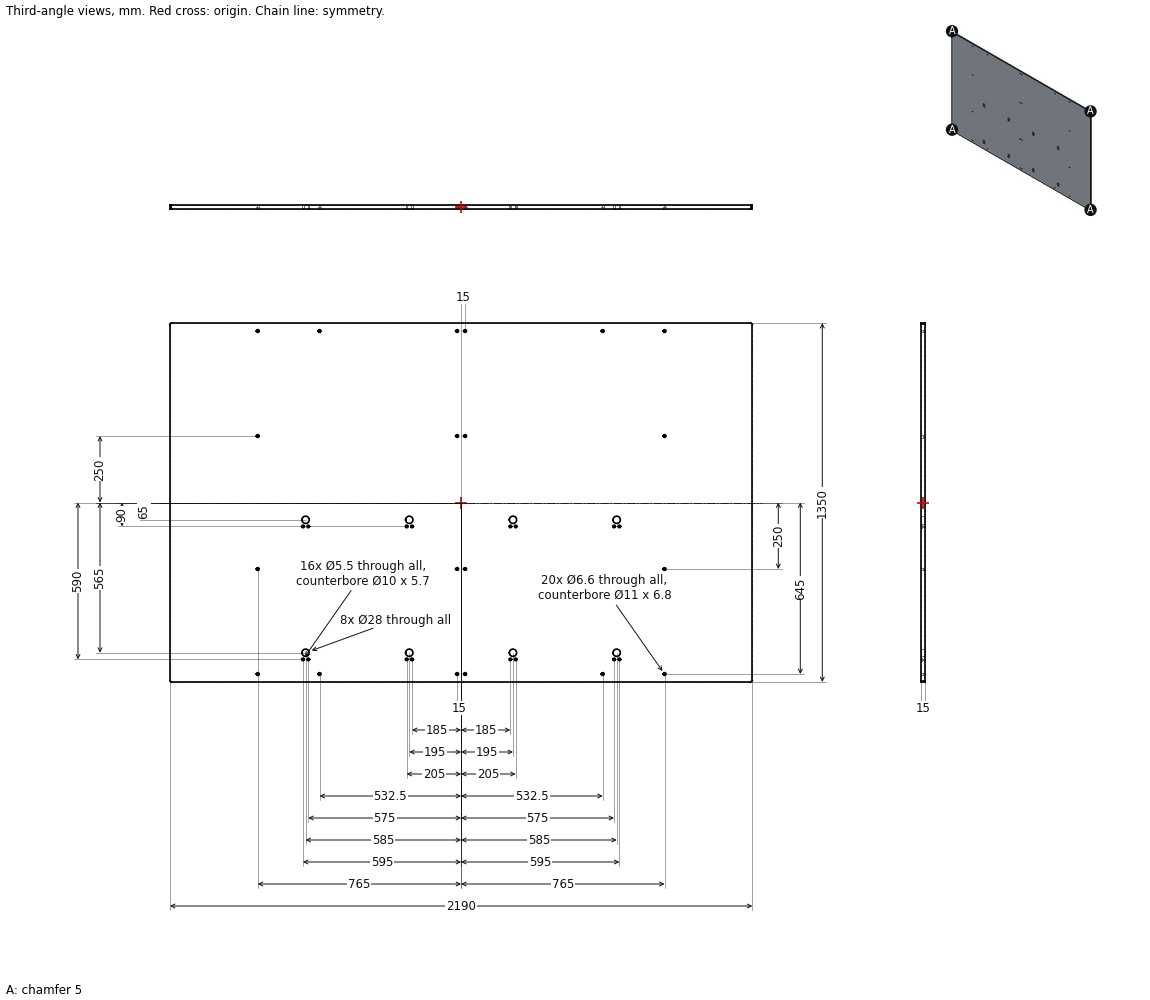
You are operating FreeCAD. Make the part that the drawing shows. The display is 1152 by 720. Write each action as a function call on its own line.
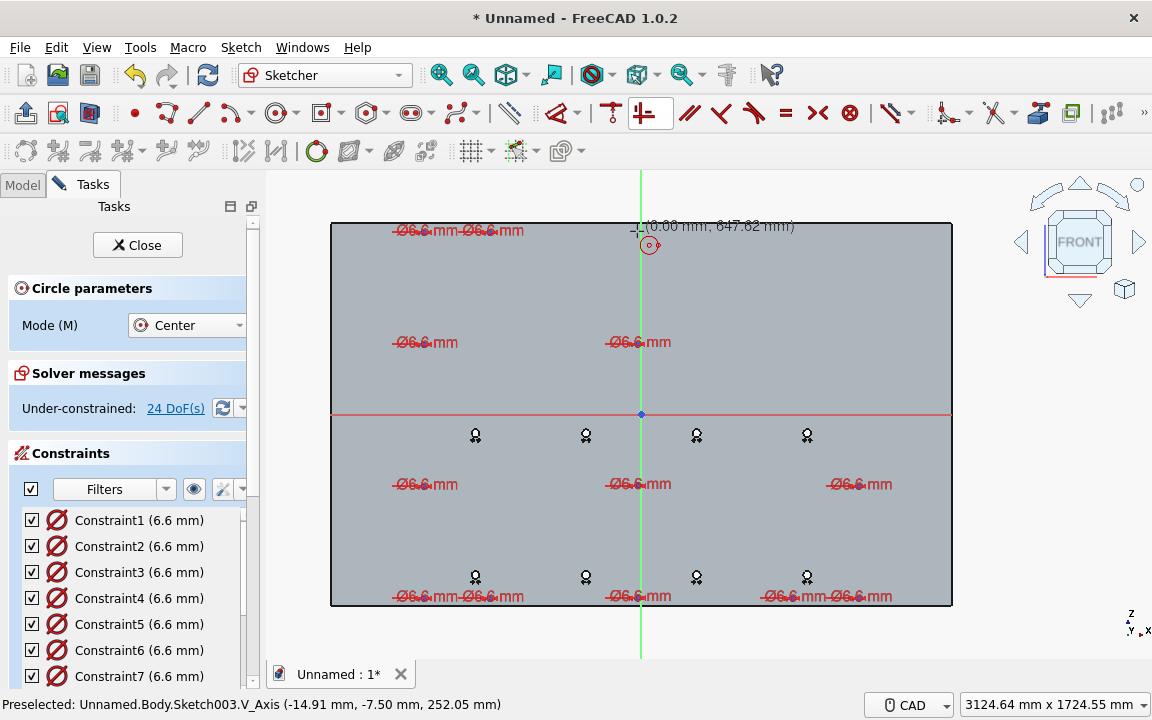
scroll(637, 232, up, 7)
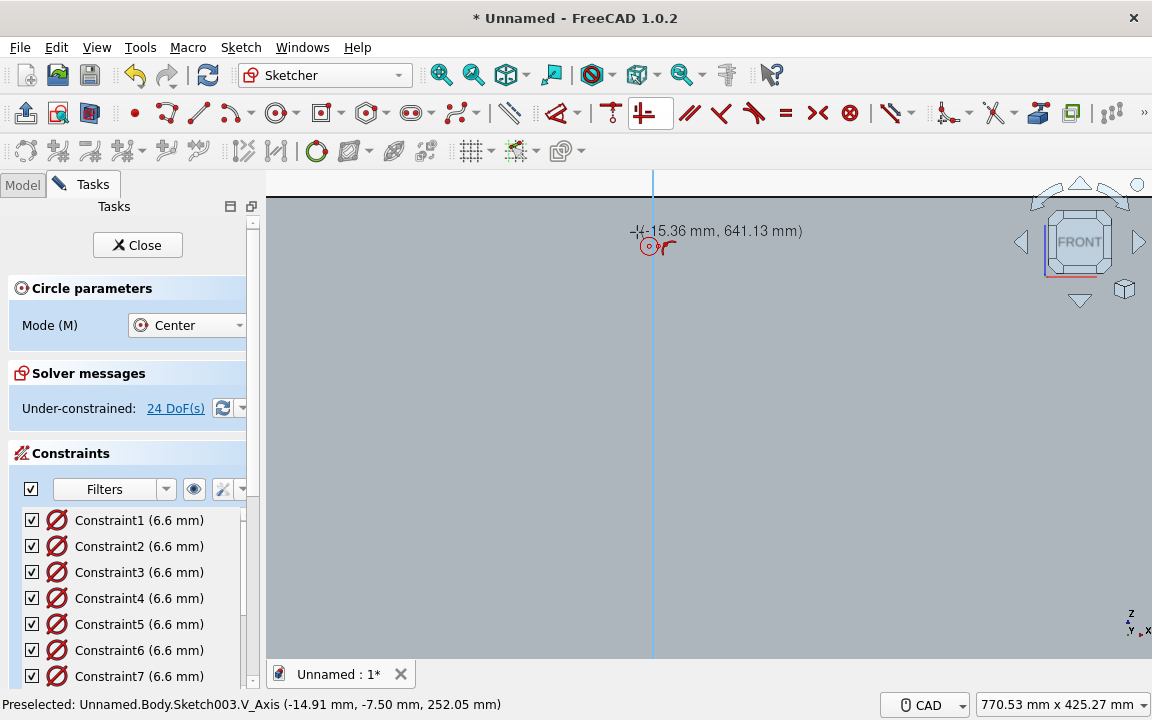
click(636, 231)
move(639, 229)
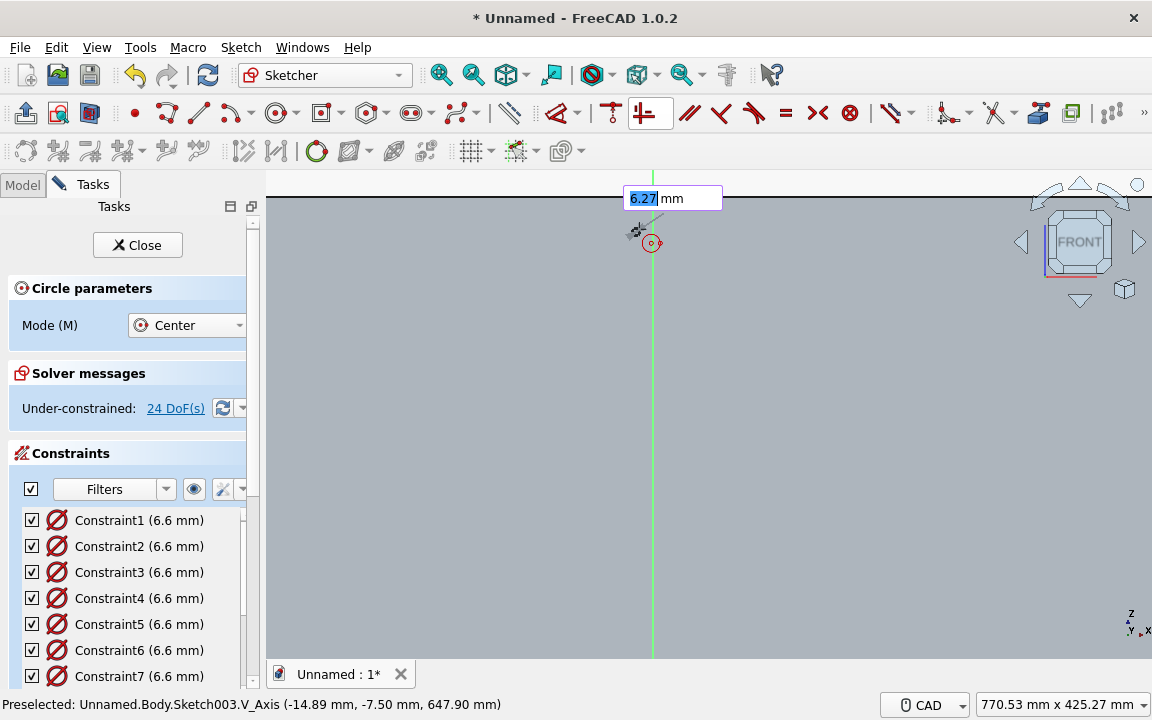
text(6.6)
key(Return)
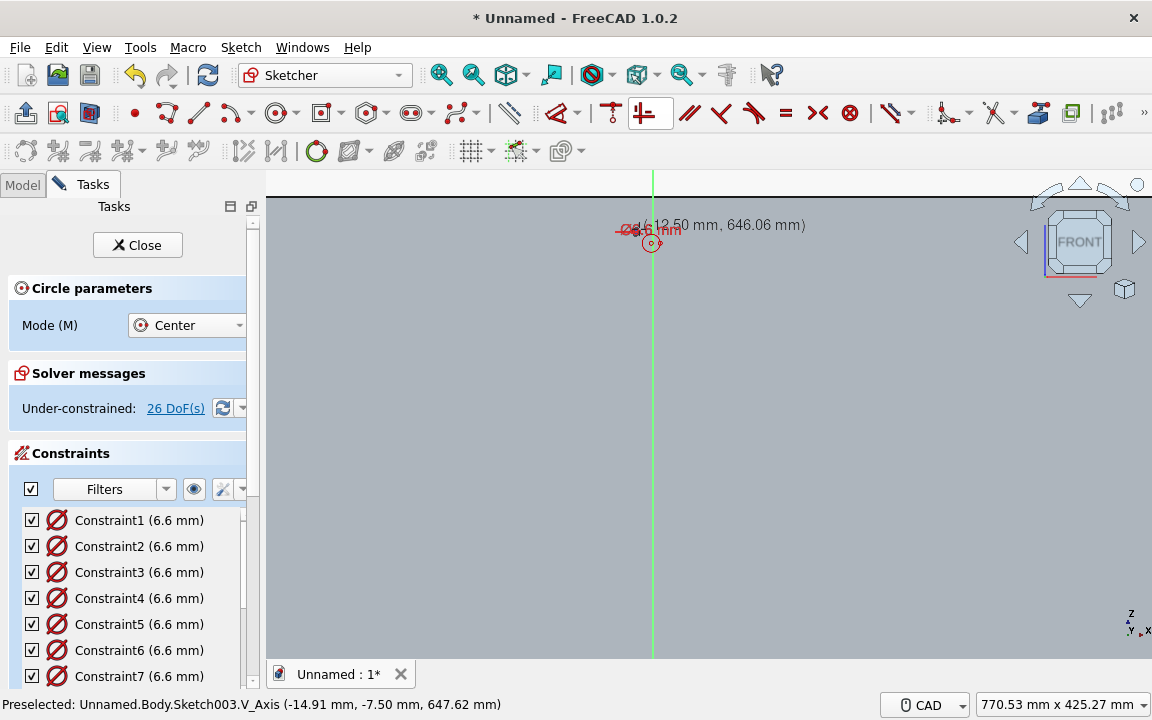
scroll(637, 273, down, 8)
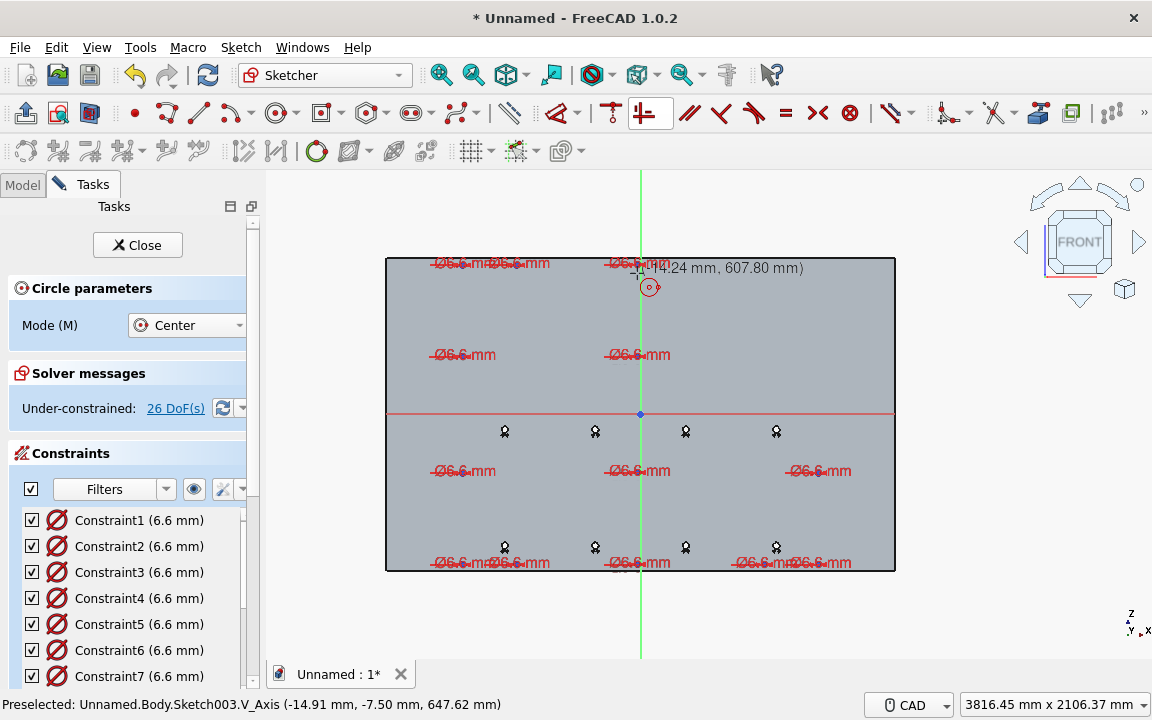
scroll(818, 356, up, 17)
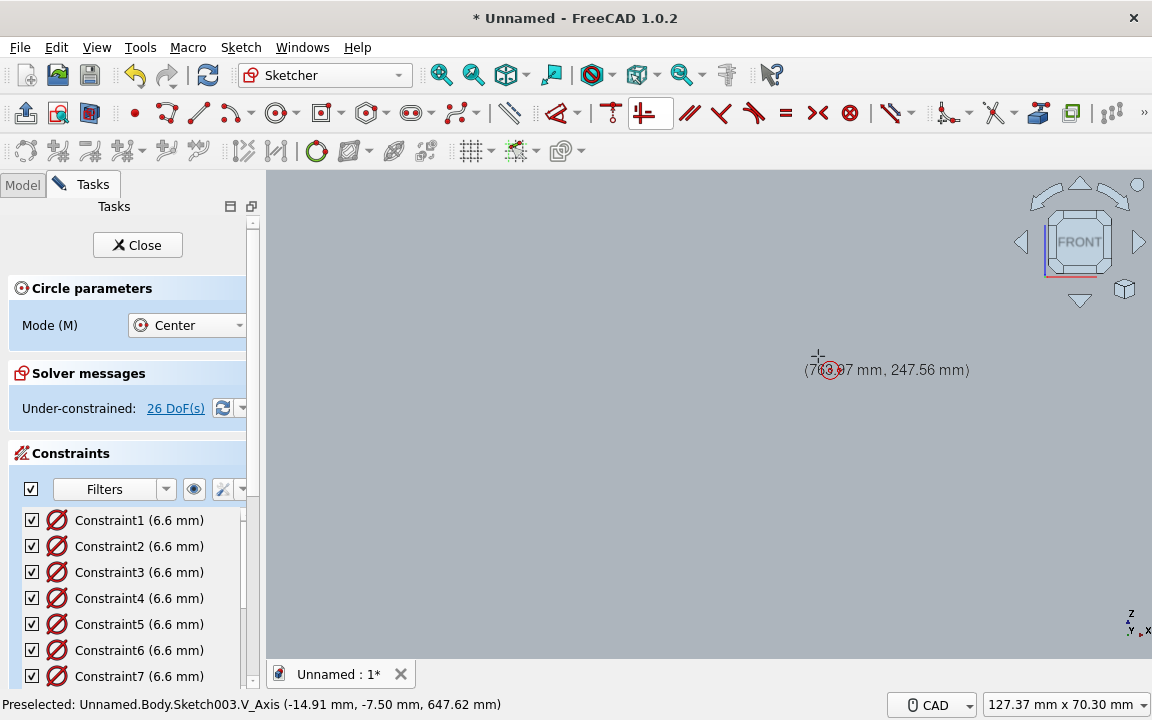
scroll(860, 343, down, 16)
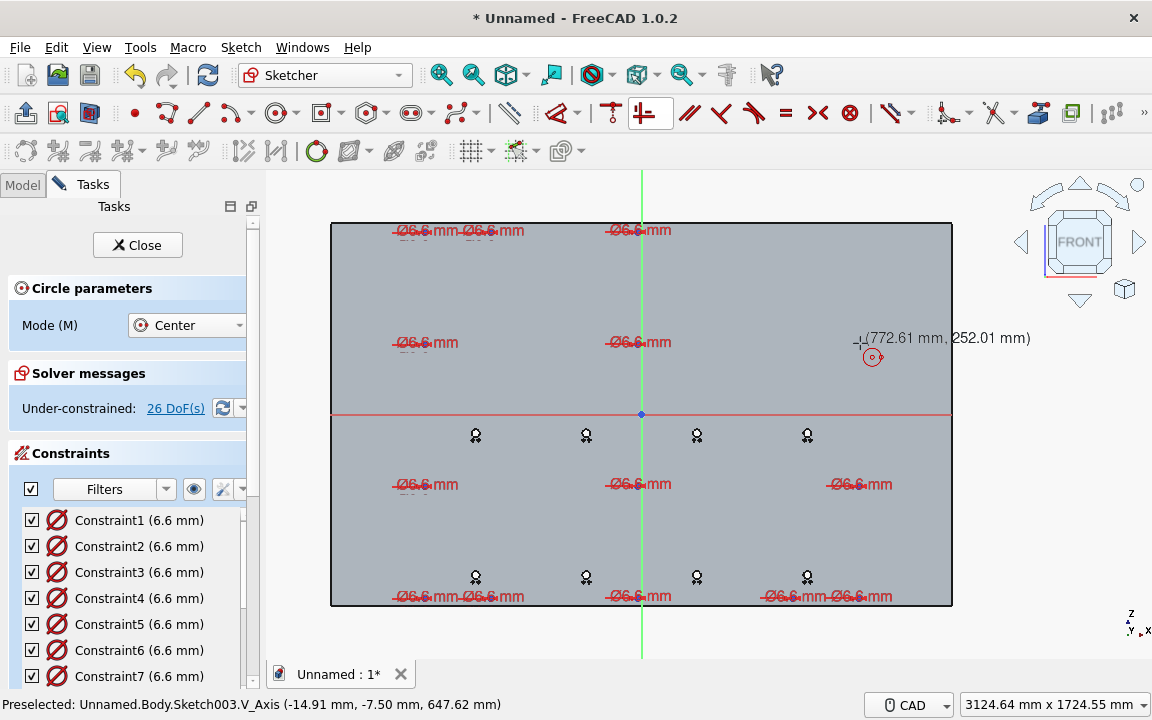
click(858, 344)
move(859, 343)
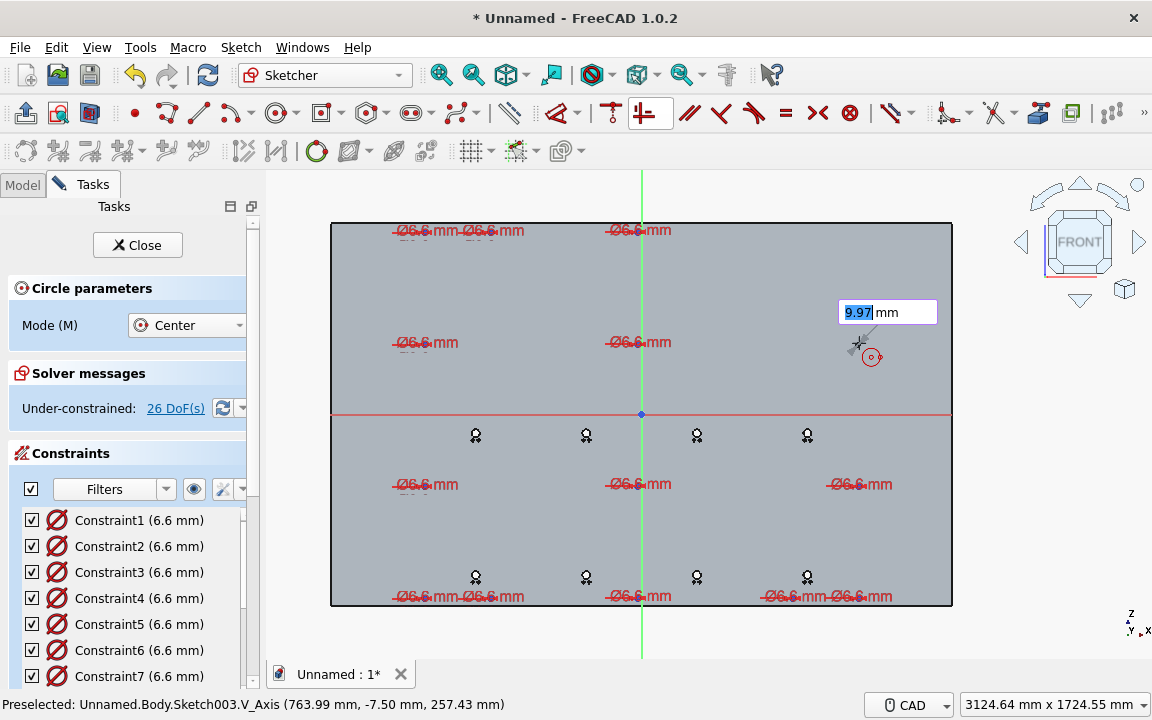
text(6.6)
key(Return)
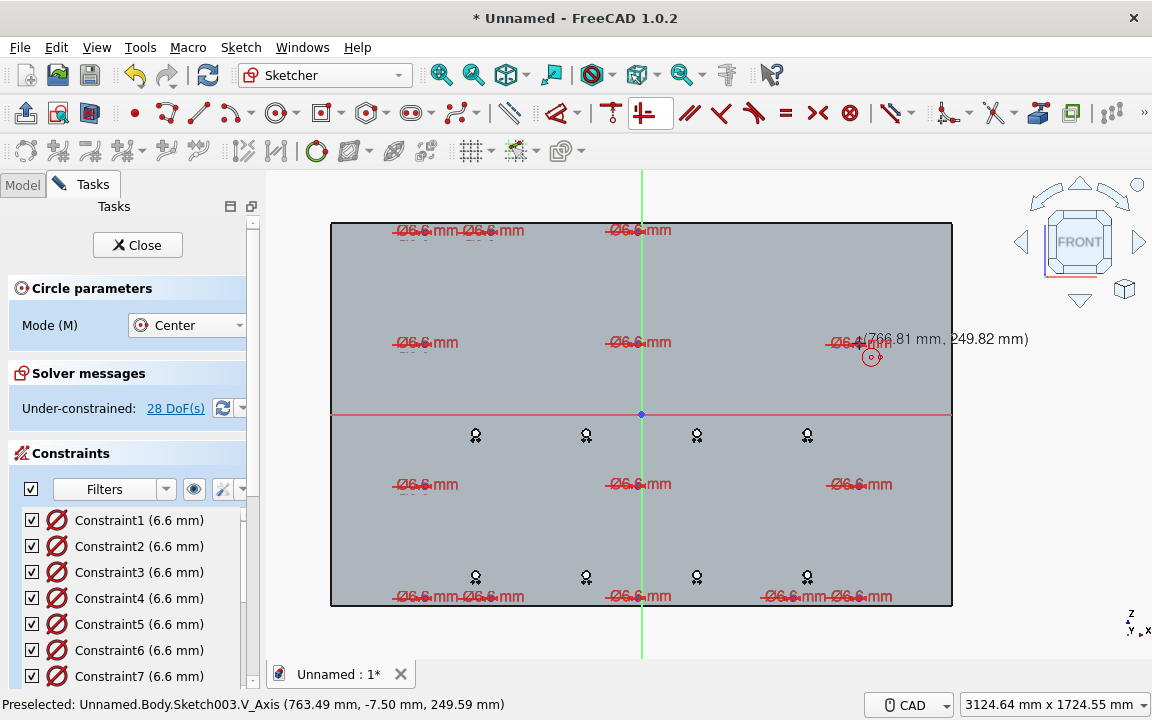
scroll(793, 232, up, 16)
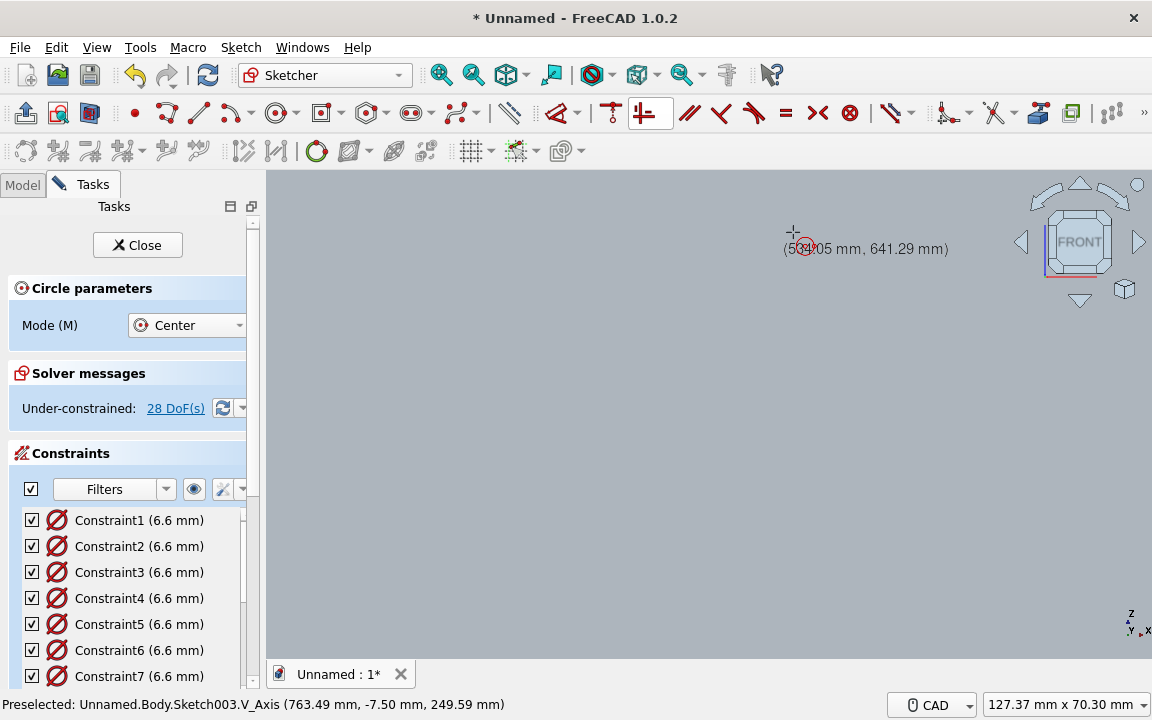
scroll(792, 232, down, 16)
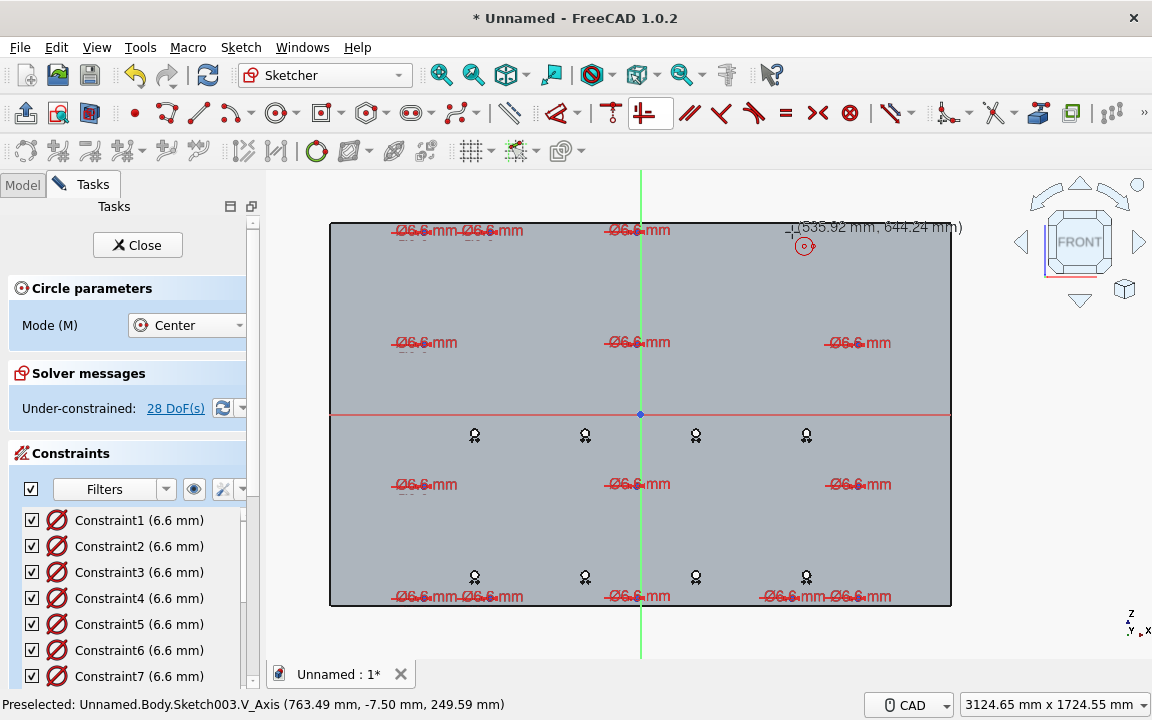
click(792, 232)
move(792, 231)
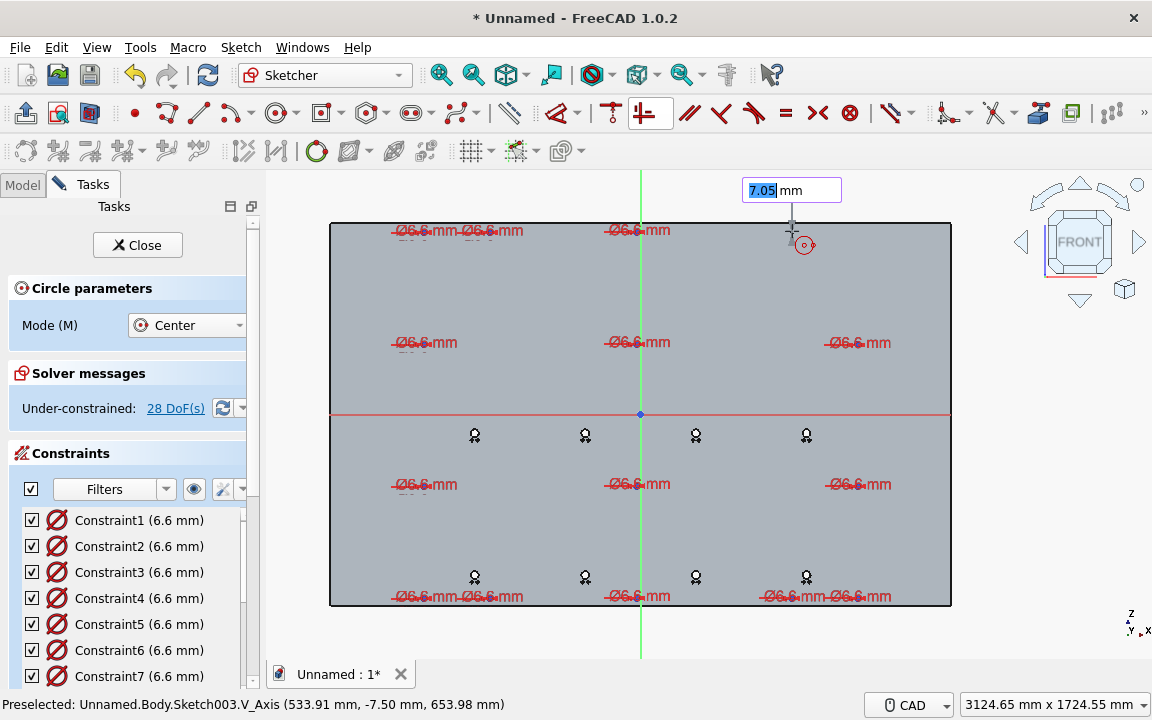
text(6.6)
key(Return)